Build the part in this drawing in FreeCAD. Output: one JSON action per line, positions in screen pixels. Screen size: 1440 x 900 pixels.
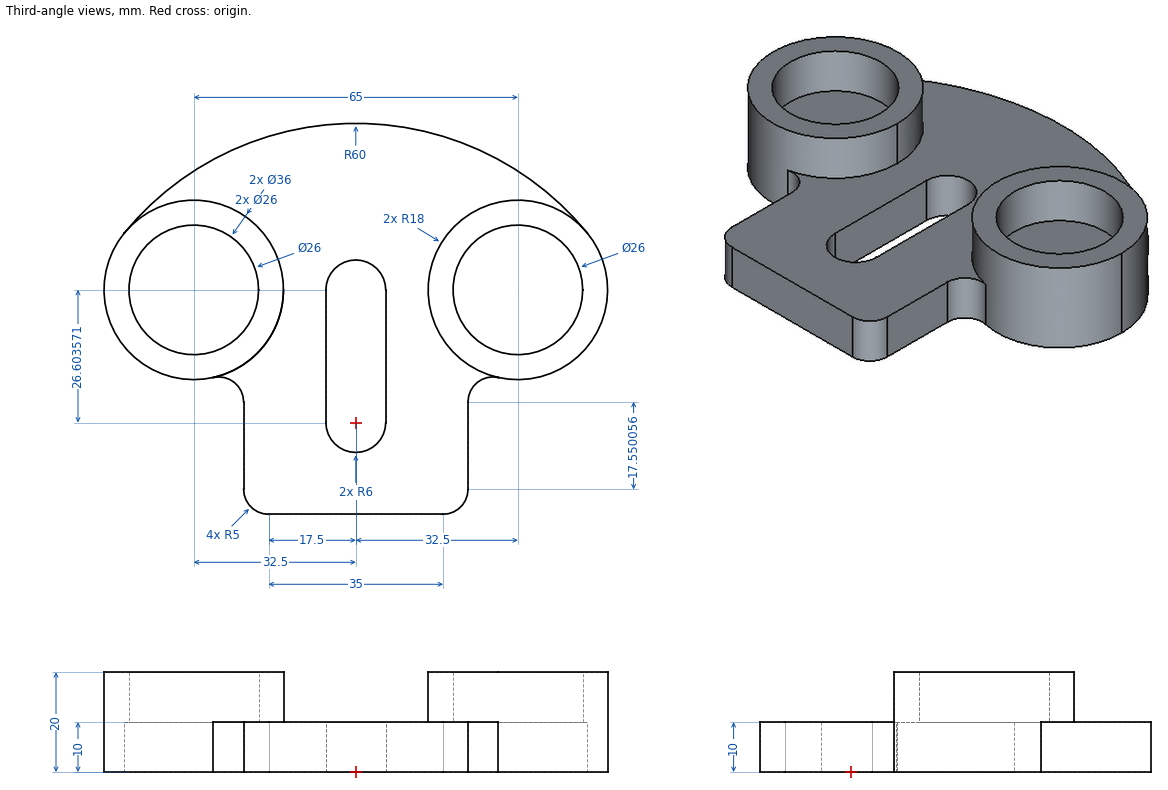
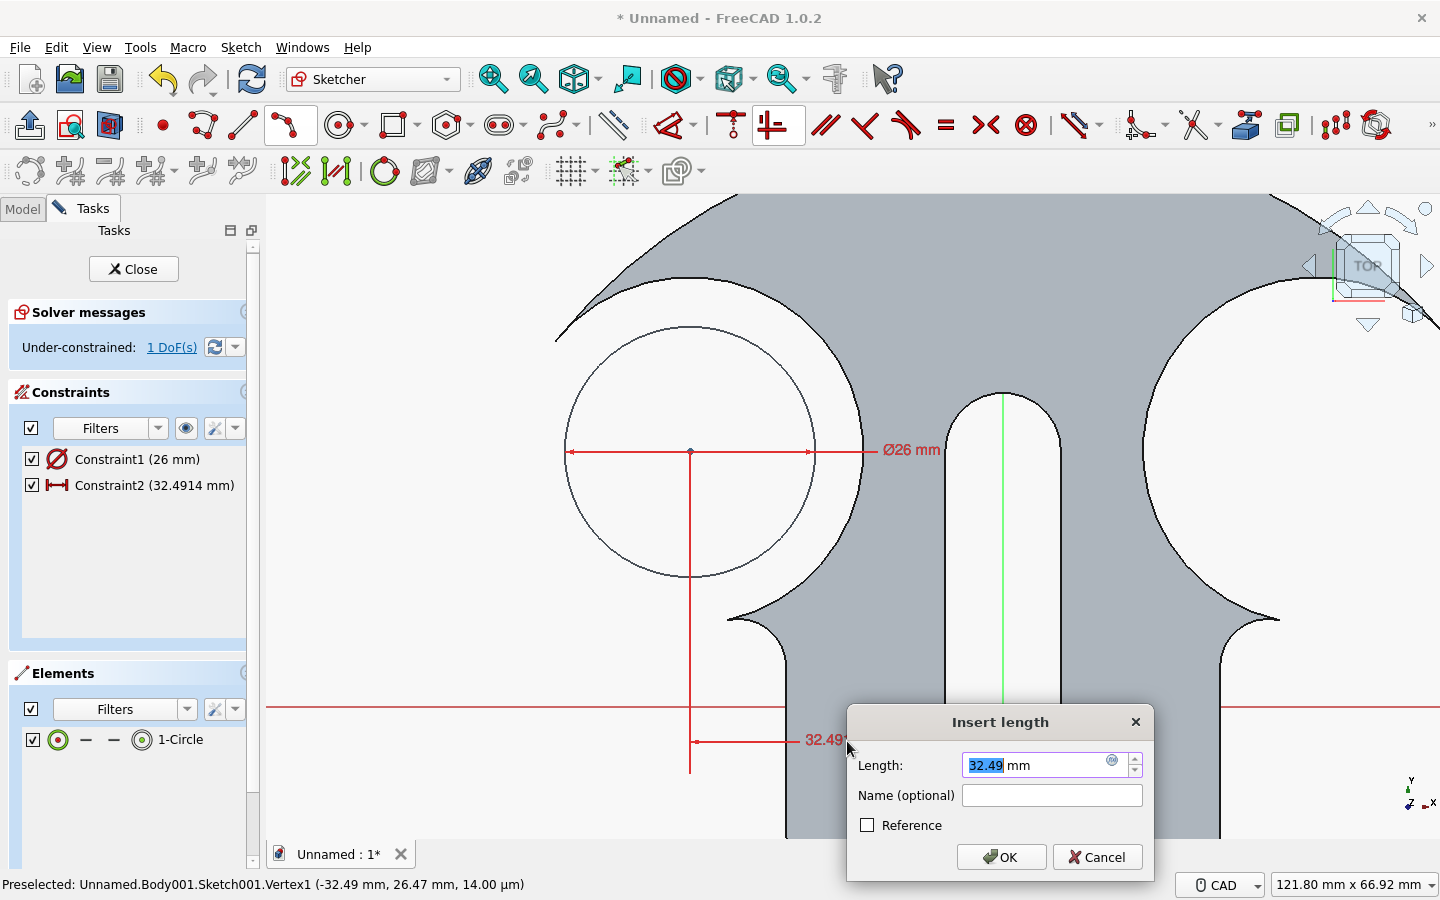
{"action": "type", "text": "32.5"}
{"action": "key", "text": "Return"}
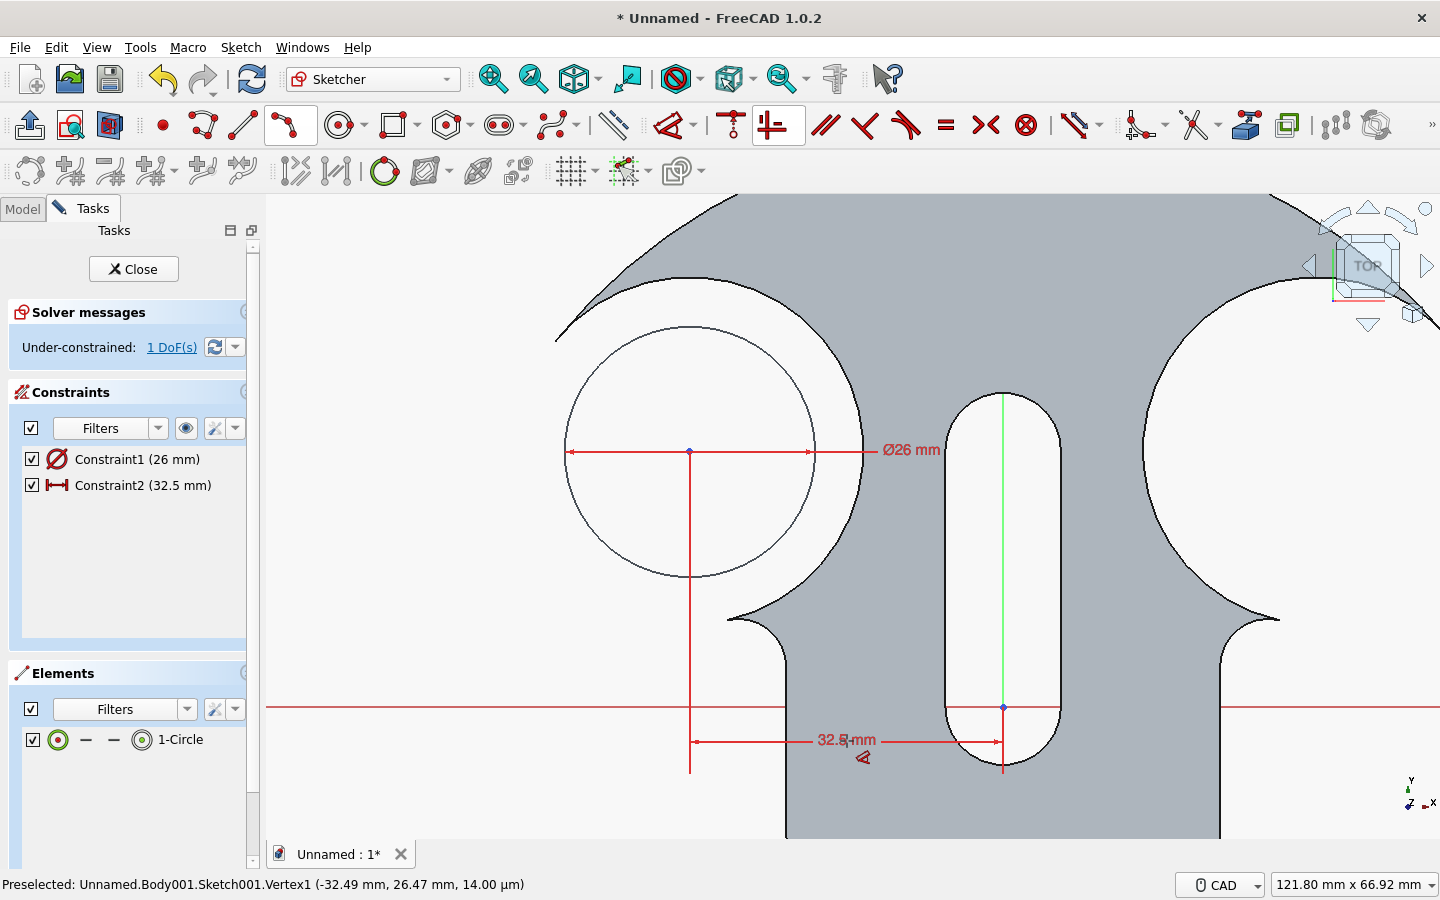
{"action": "left_click", "coordinate": [690, 452]}
{"action": "left_click", "coordinate": [1037, 580]}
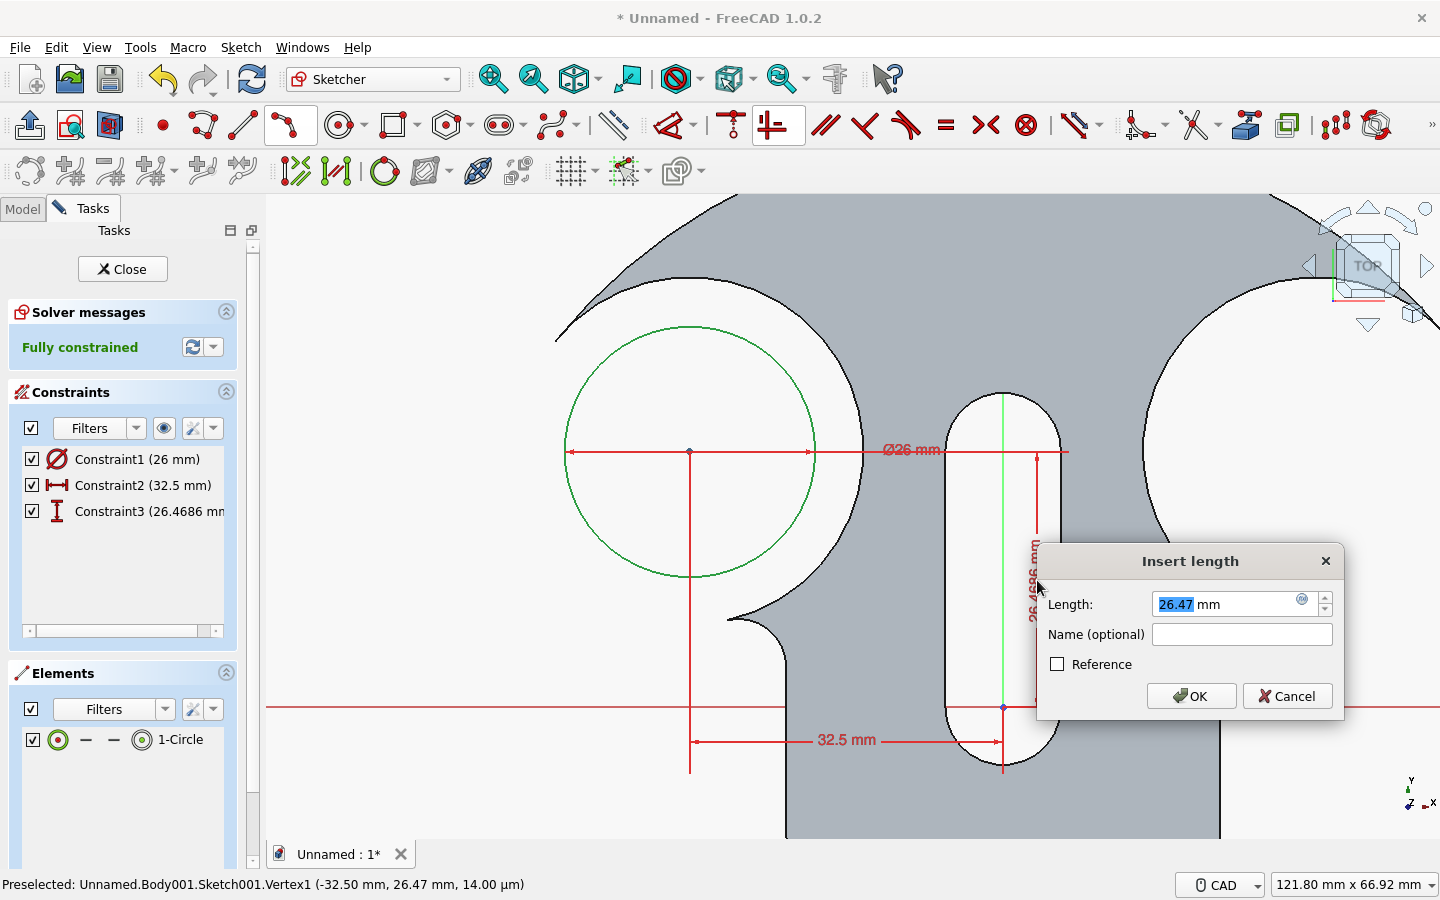
{"action": "type", "text": "26.603571"}
{"action": "key", "text": "Return"}
{"action": "key", "text": "Escape"}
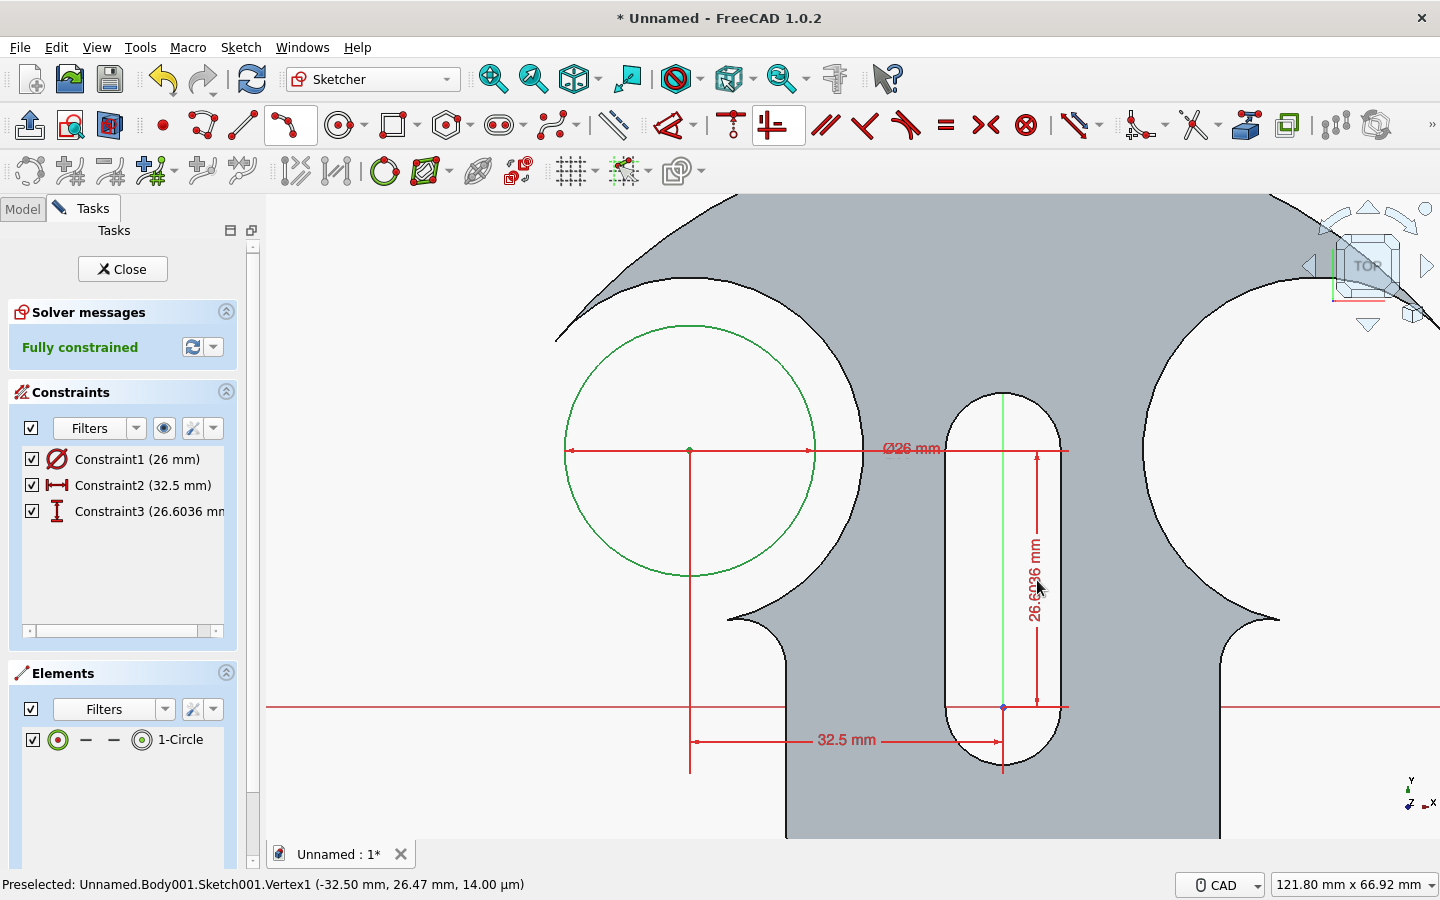
{"action": "left_click", "coordinate": [123, 269]}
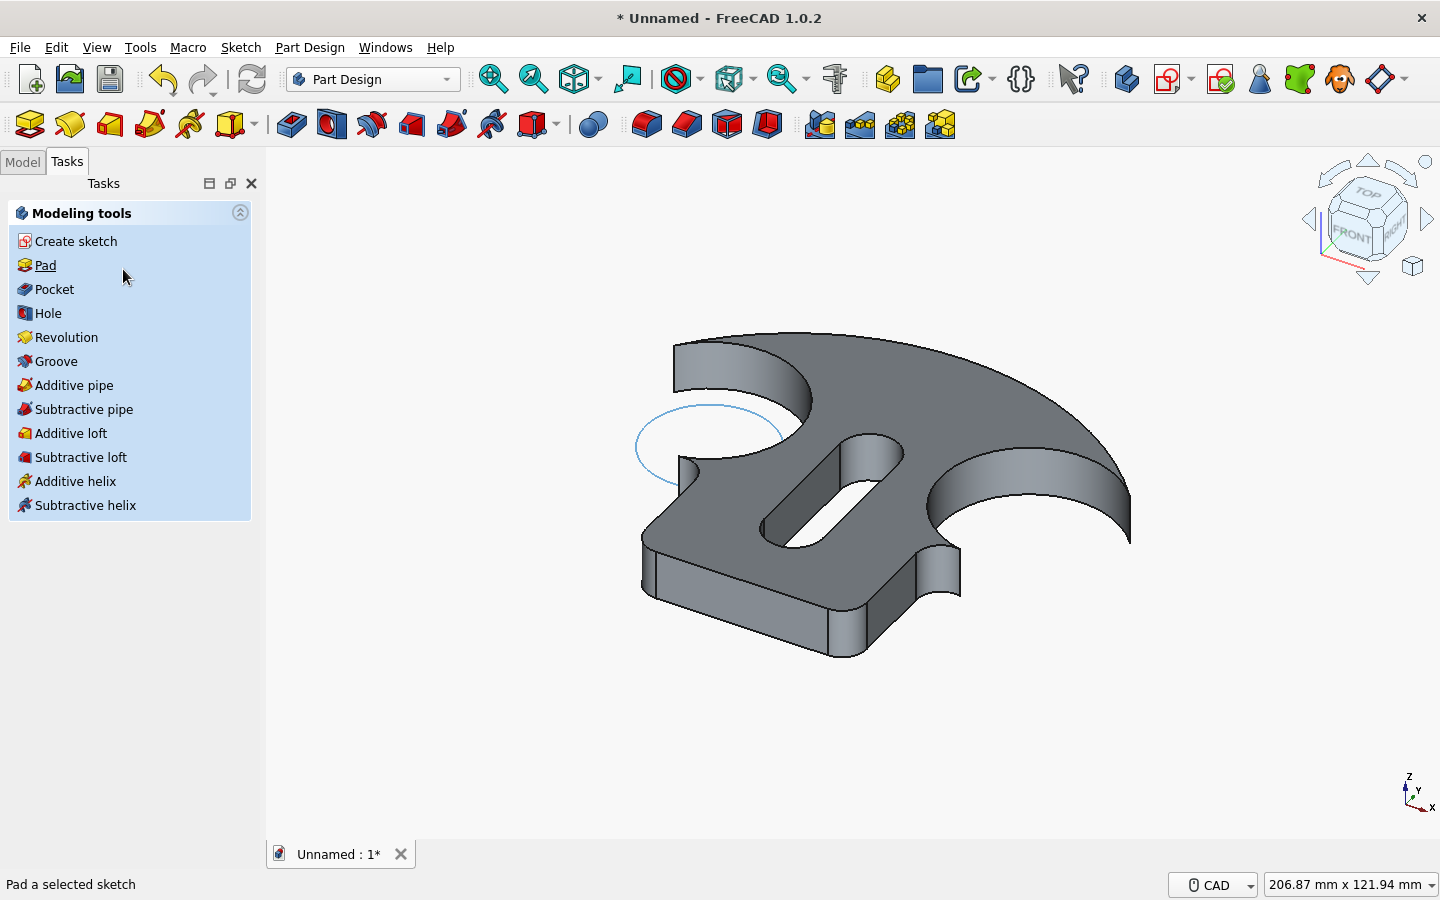
{"action": "left_click", "coordinate": [30, 124]}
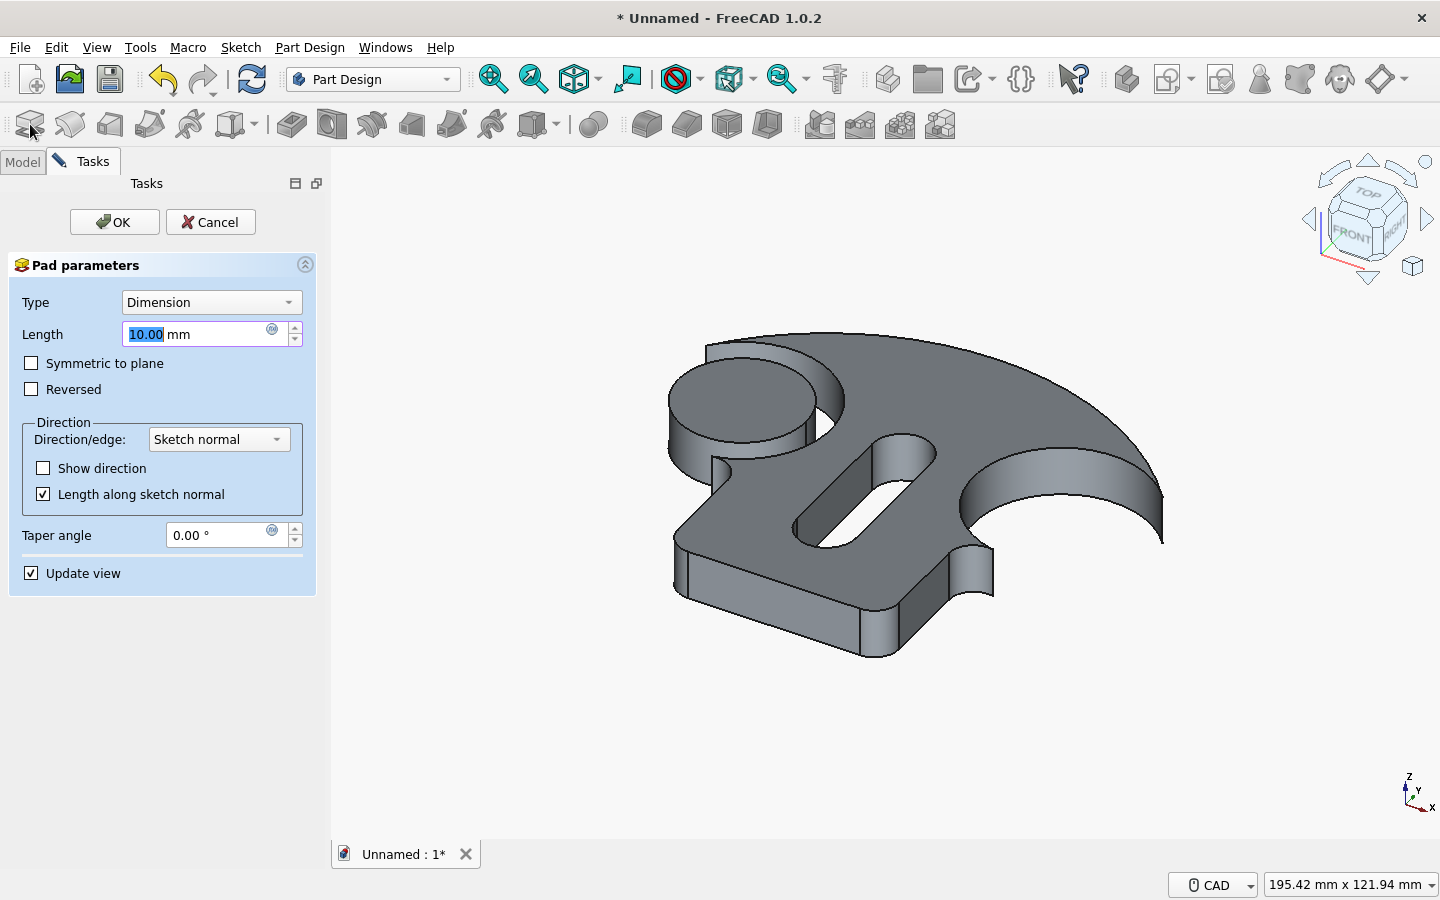
{"action": "type", "text": "10"}
{"action": "key", "text": "Tab"}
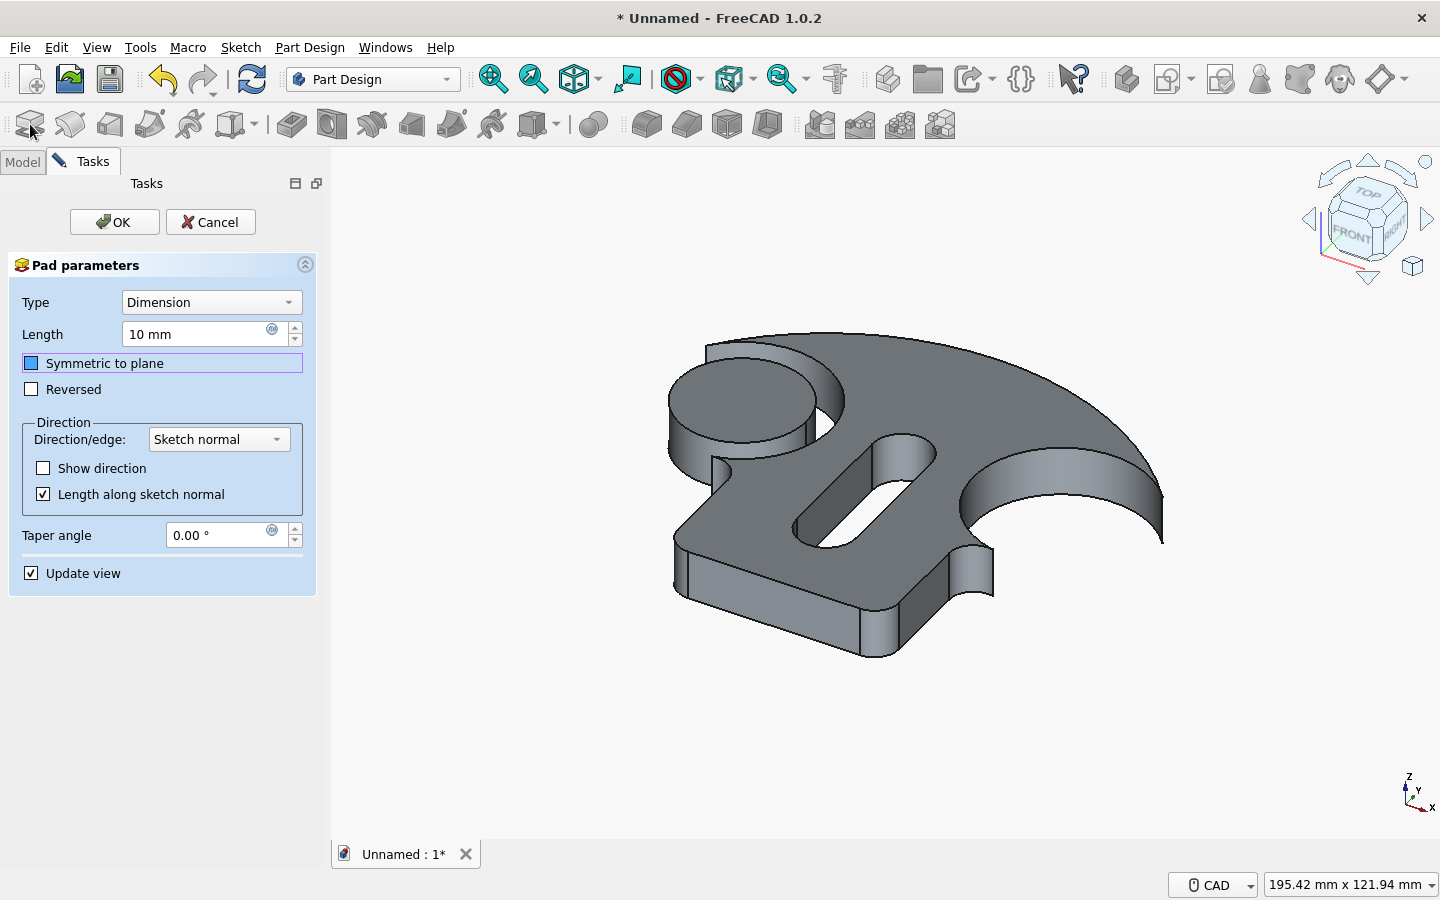
{"action": "left_click", "coordinate": [115, 222]}